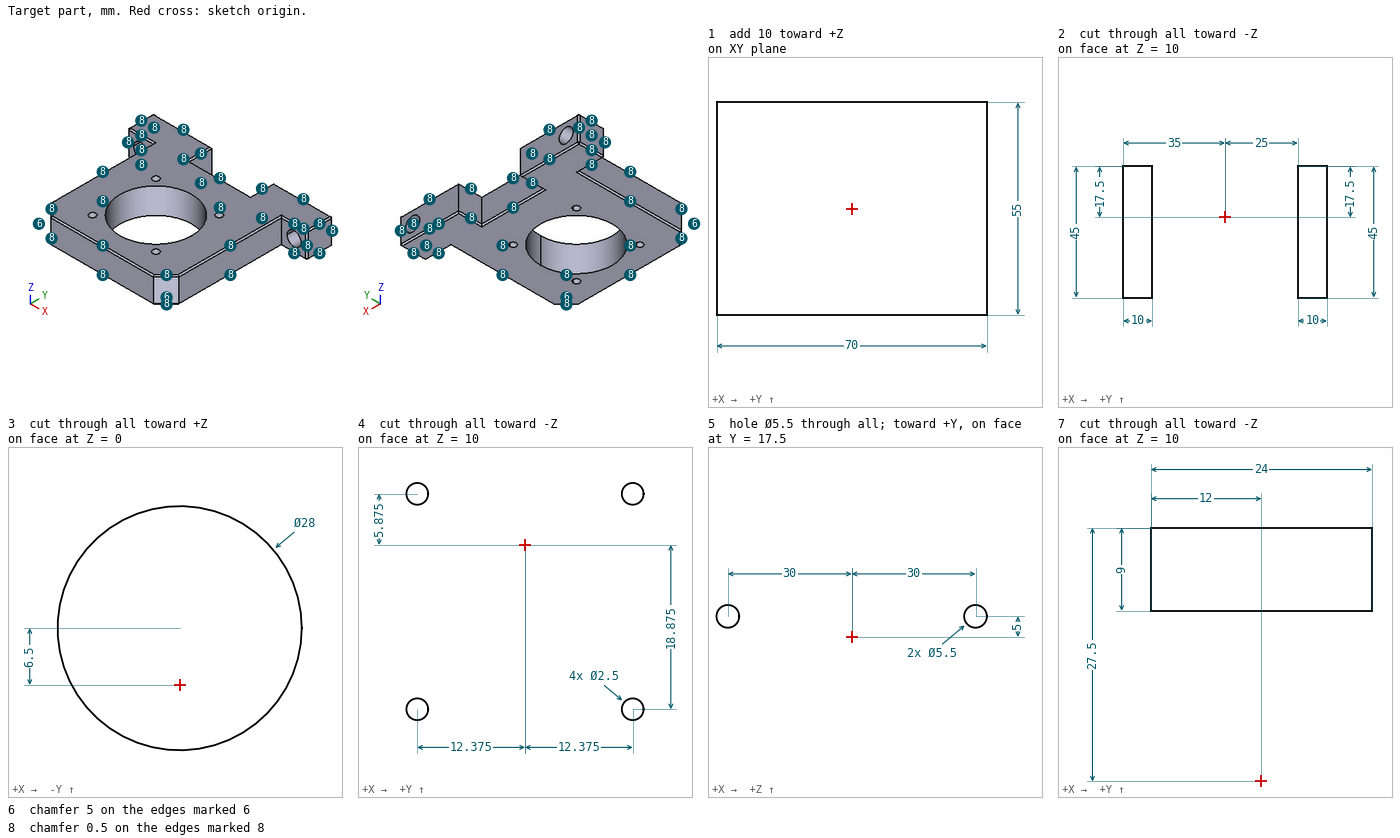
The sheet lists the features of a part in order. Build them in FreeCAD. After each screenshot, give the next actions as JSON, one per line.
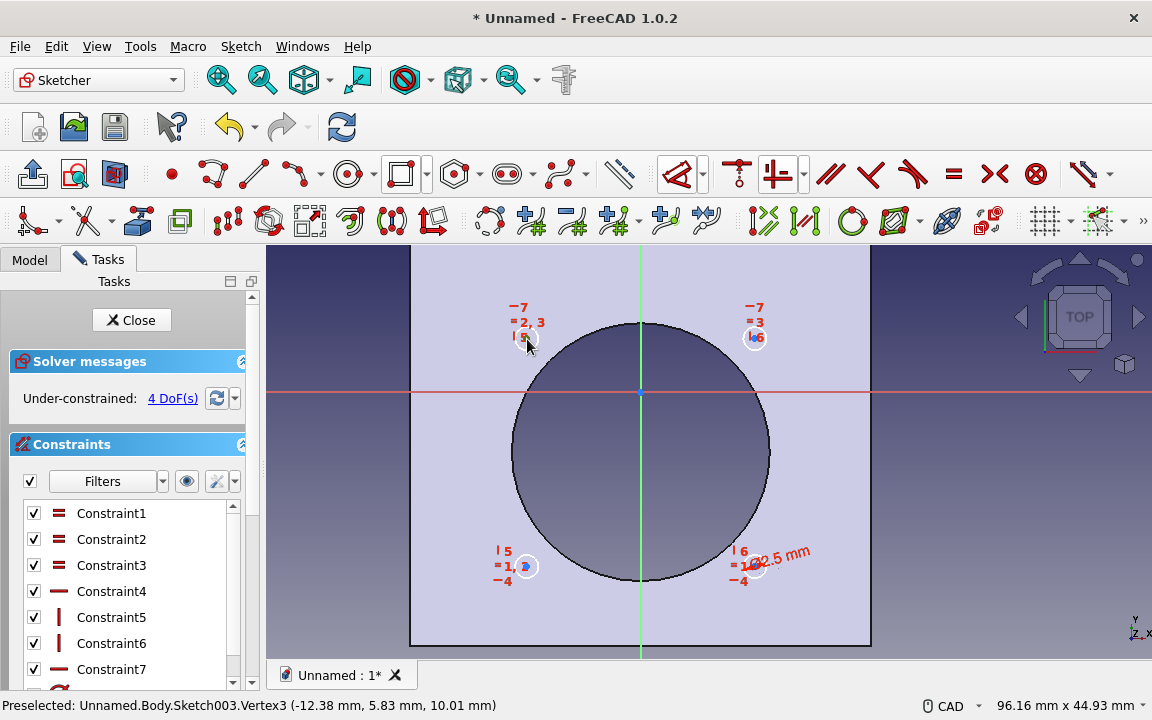
{"action": "key", "text": "i"}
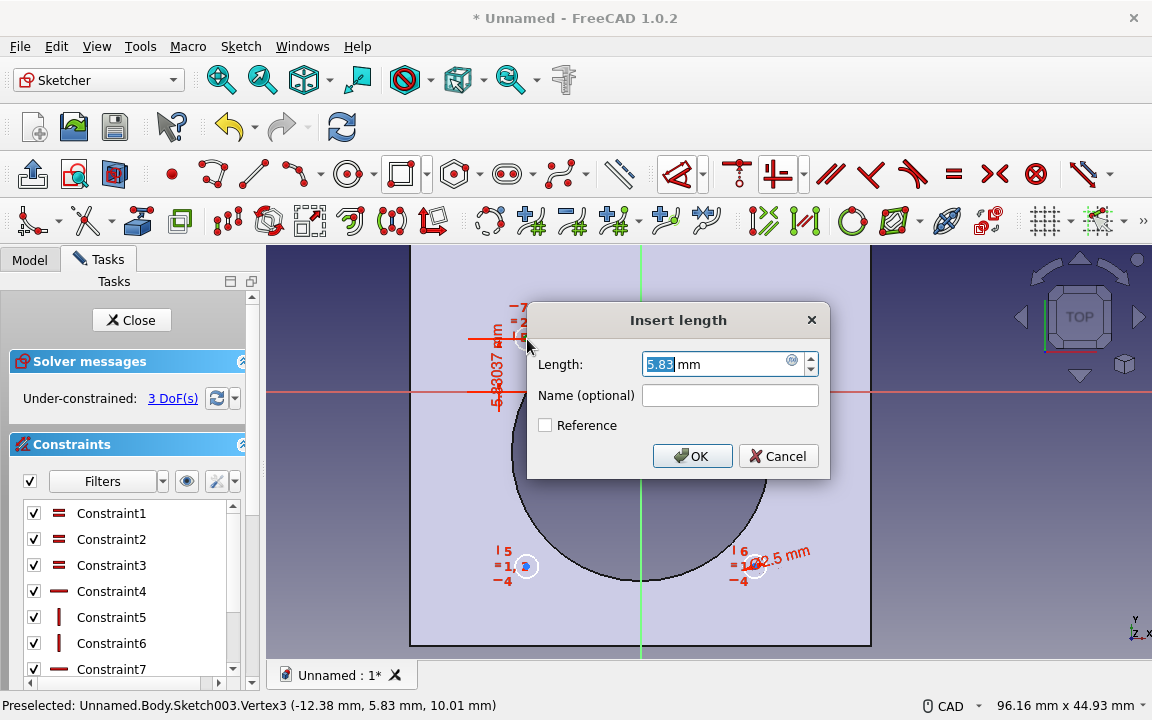
{"action": "type", "text": "5.875"}
{"action": "key", "text": "Return"}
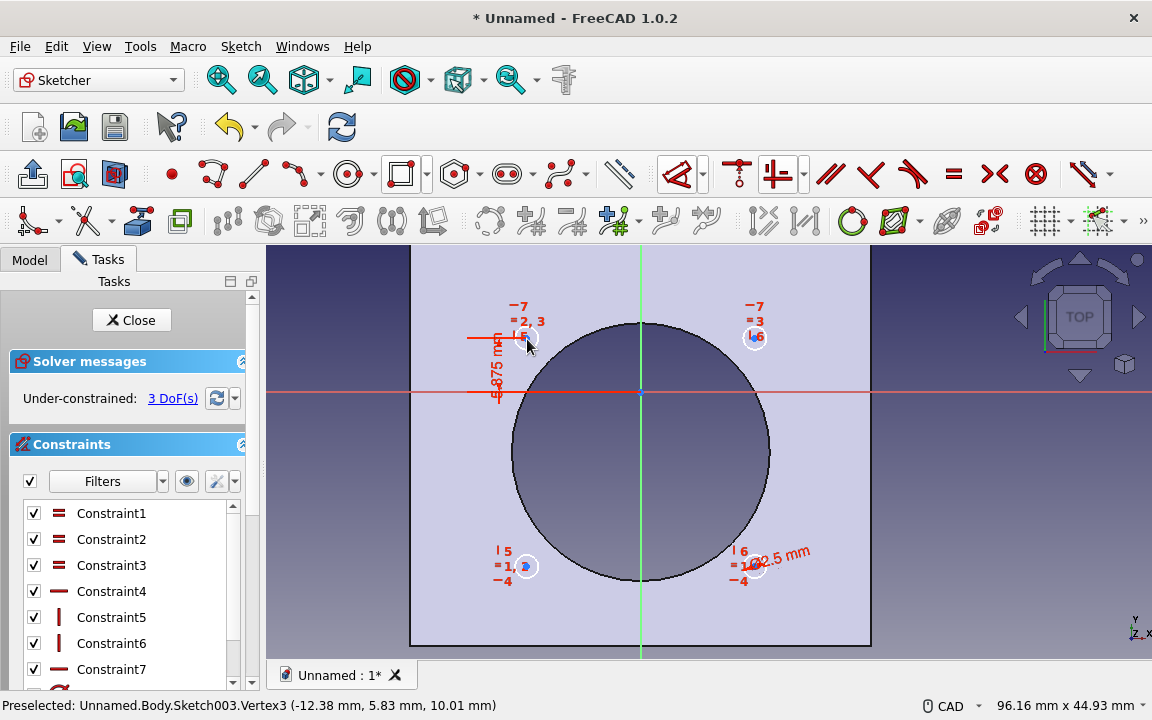
{"action": "left_click", "coordinate": [755, 567]}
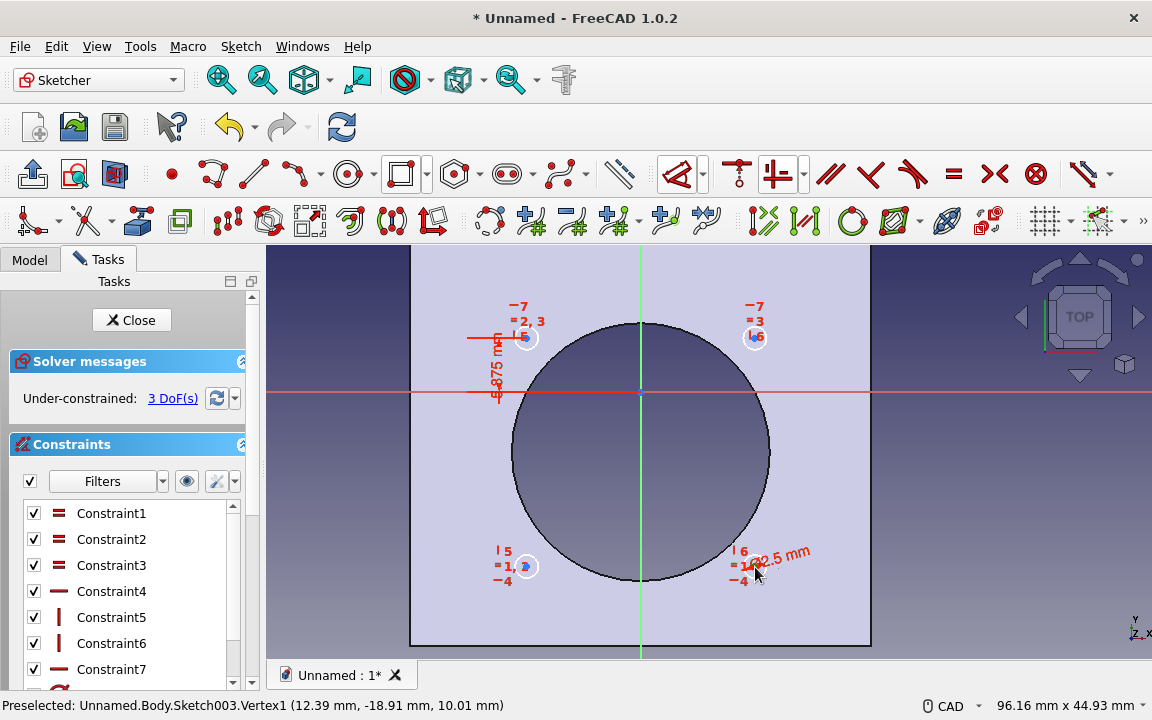
{"action": "left_click", "coordinate": [702, 174]}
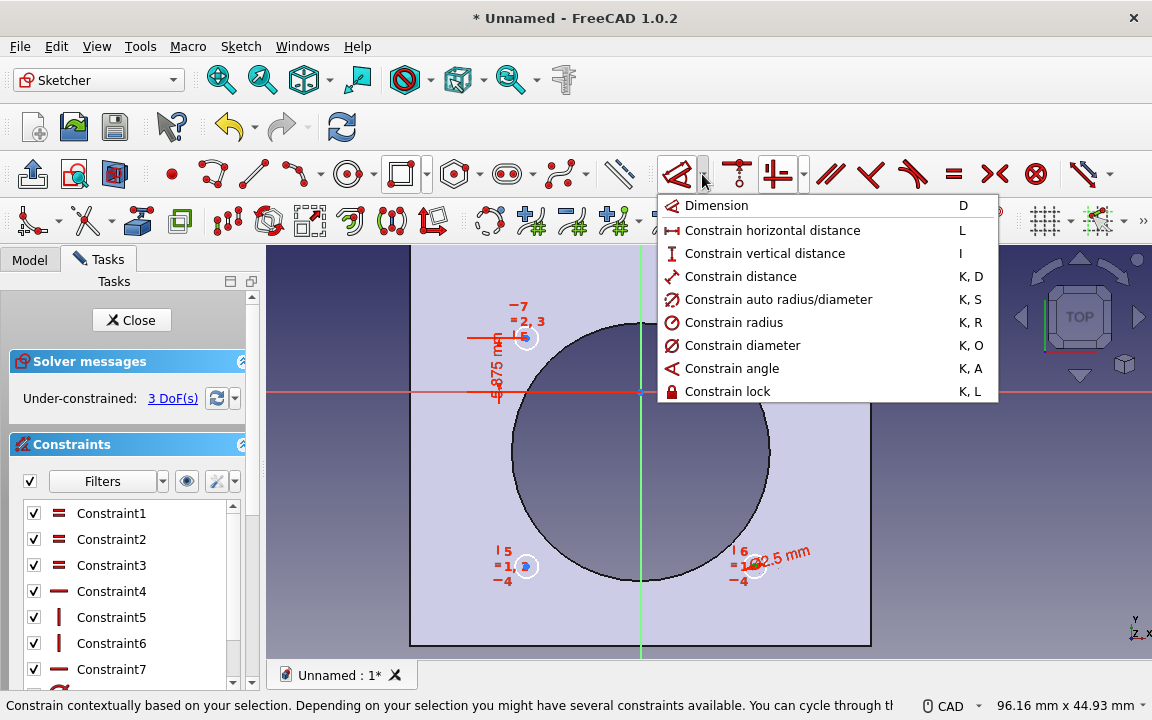
{"action": "left_click", "coordinate": [828, 230]}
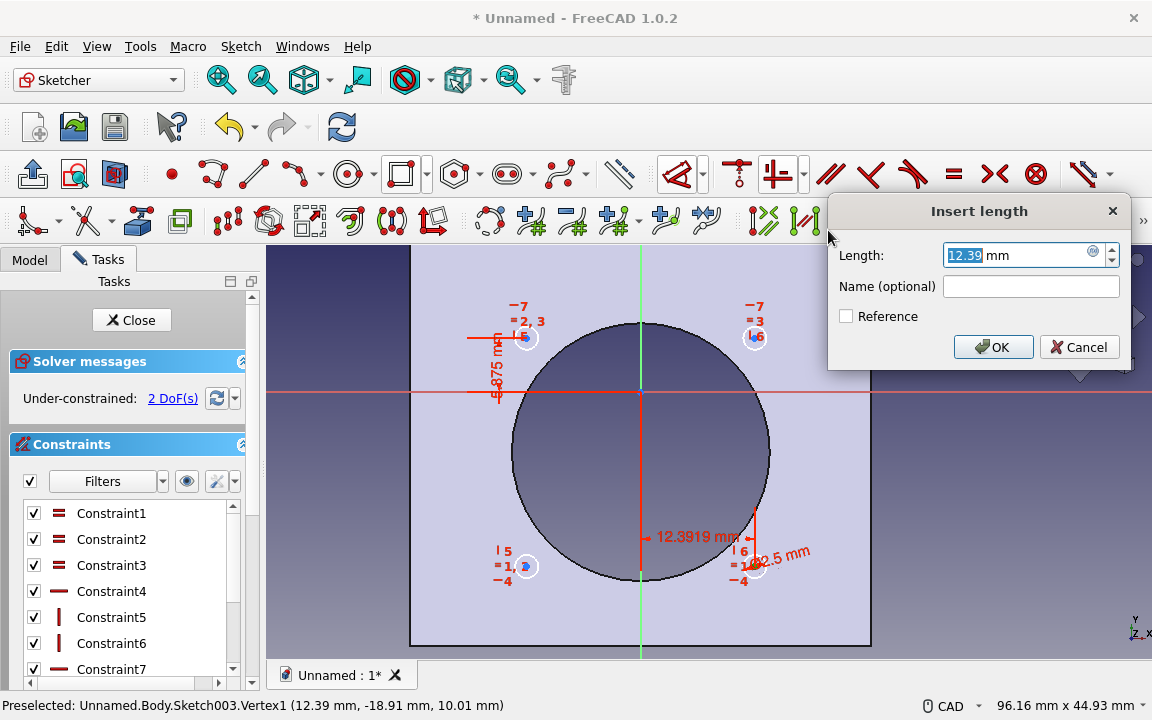
{"action": "type", "text": "12.375"}
{"action": "key", "text": "Return"}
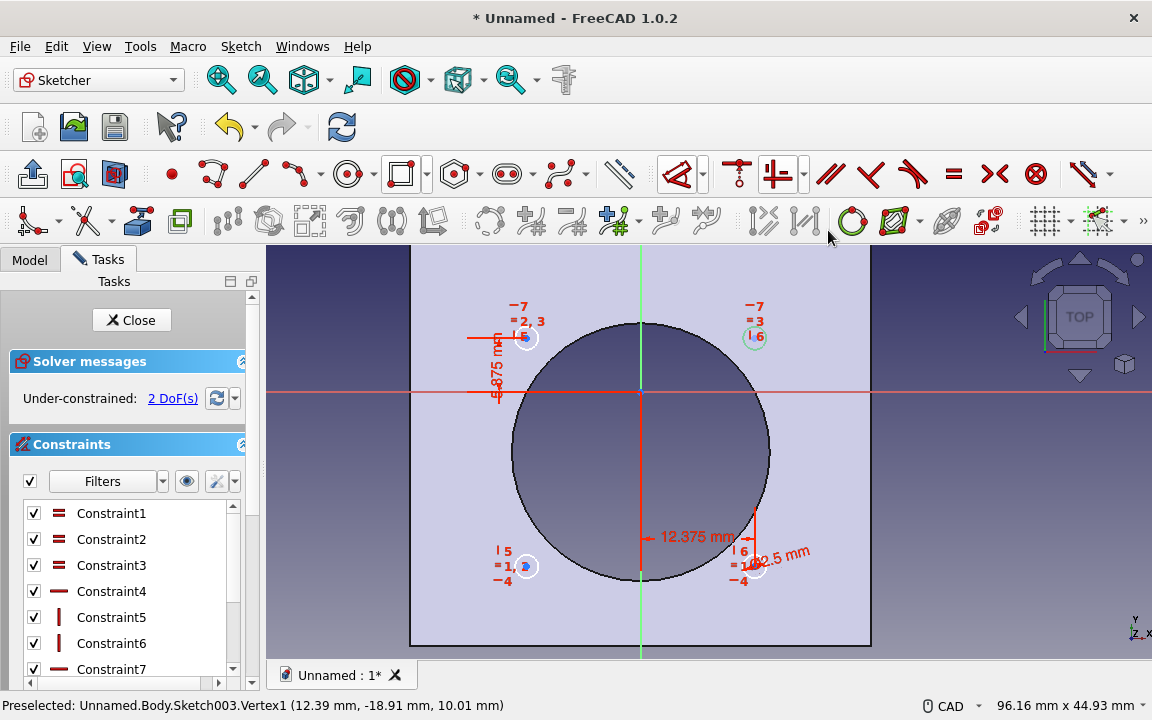
{"action": "left_click", "coordinate": [755, 567]}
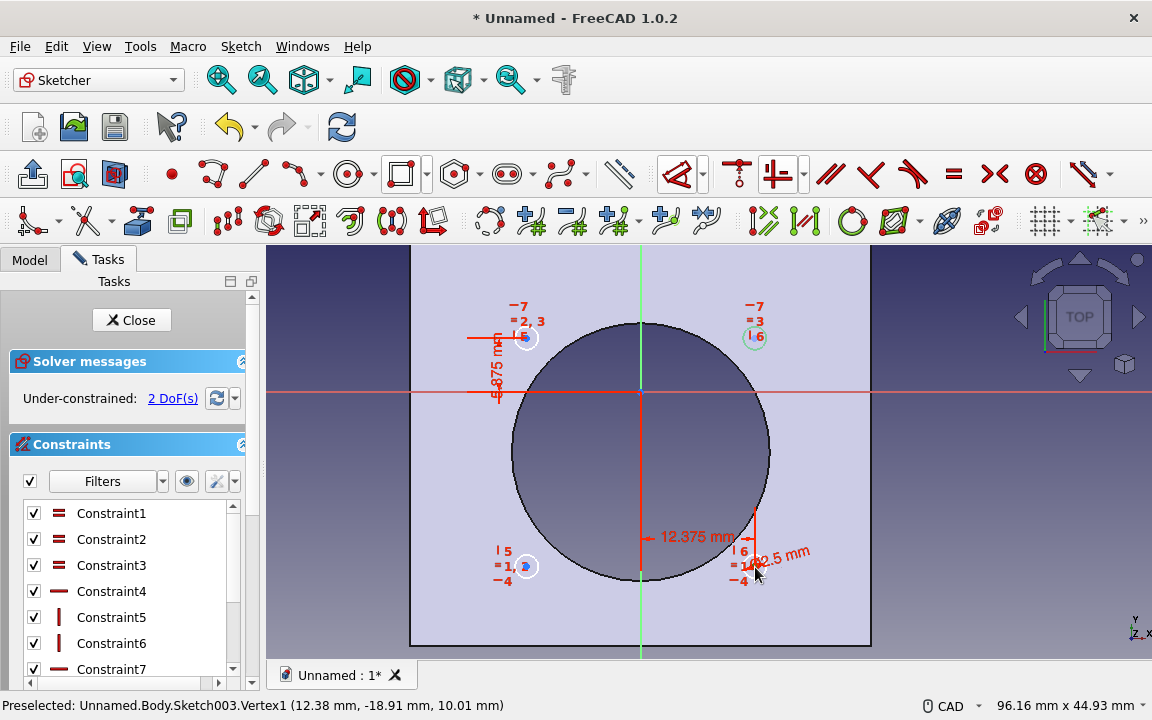
{"action": "left_click", "coordinate": [702, 174]}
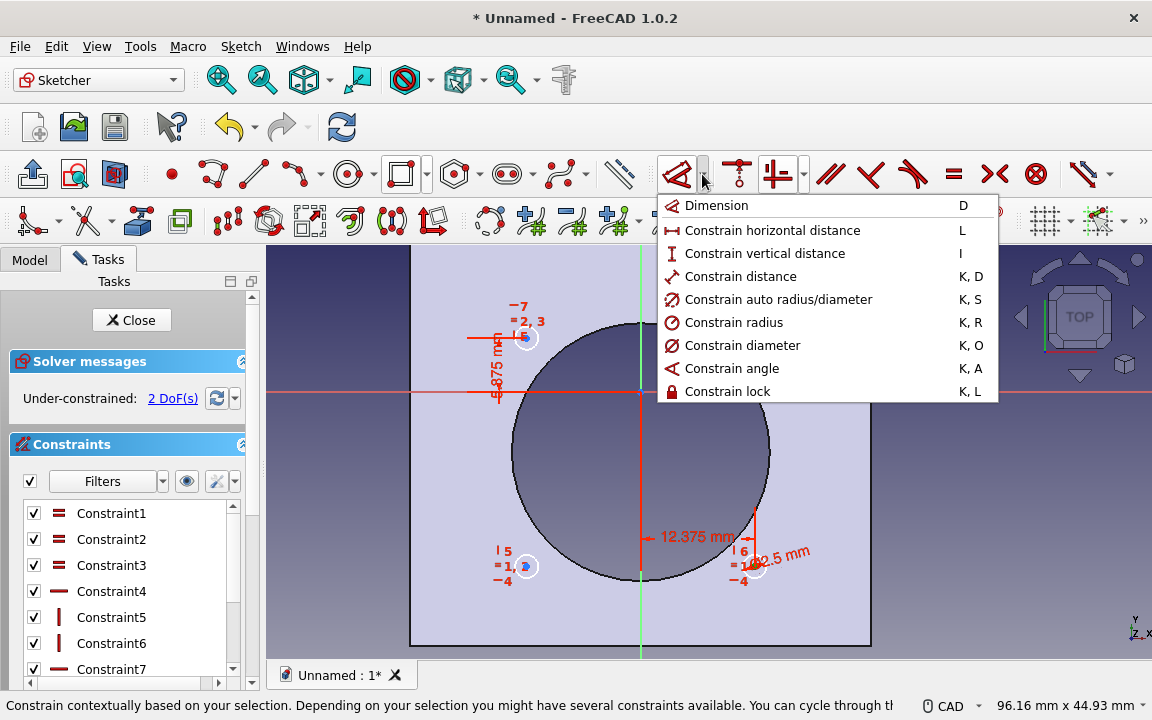
{"action": "left_click", "coordinate": [828, 254]}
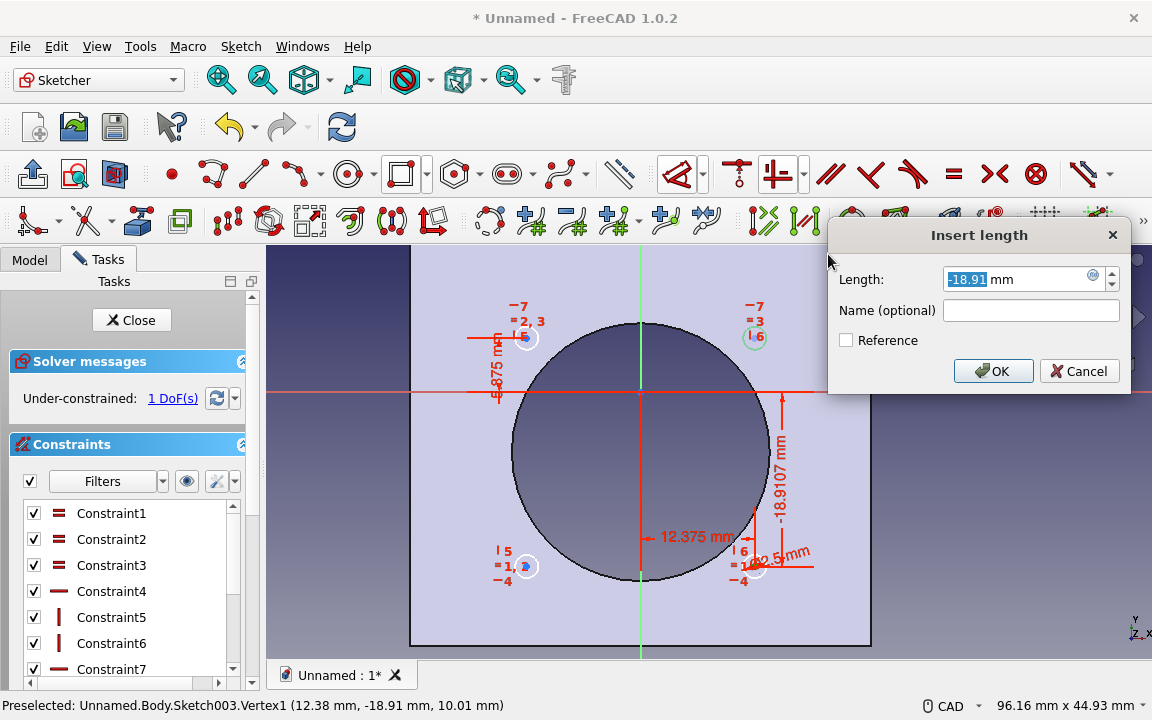
{"action": "type", "text": "-18.875"}
{"action": "key", "text": "Return"}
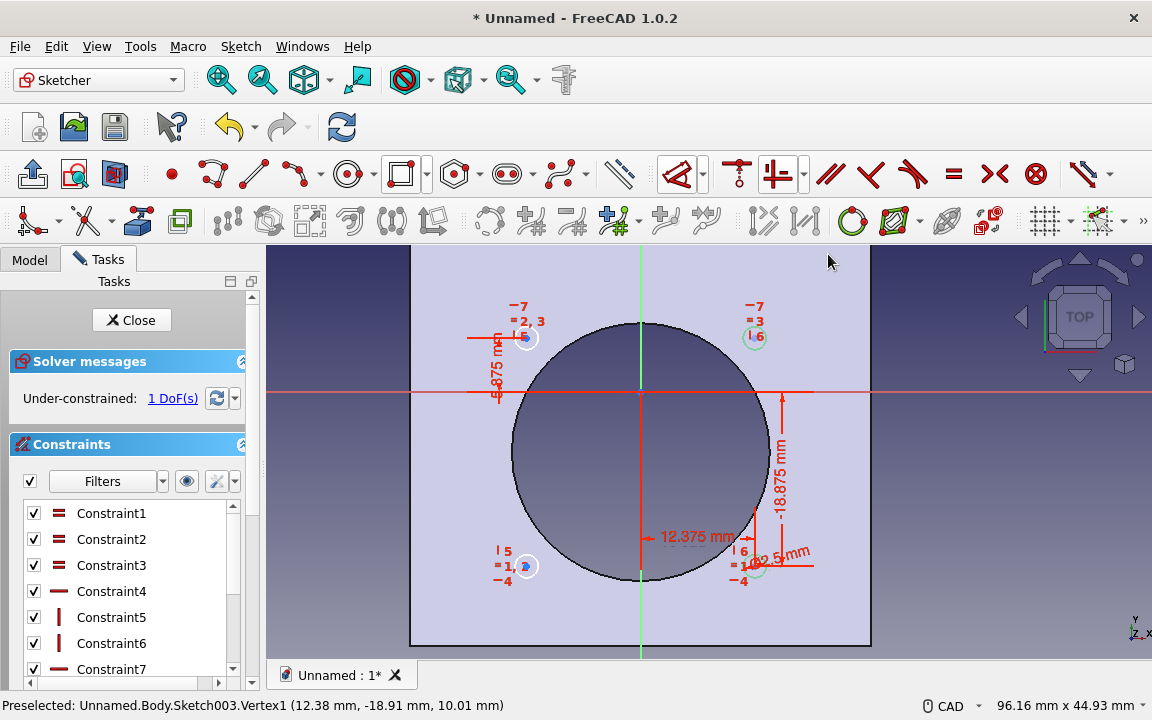
{"action": "left_click", "coordinate": [527, 566]}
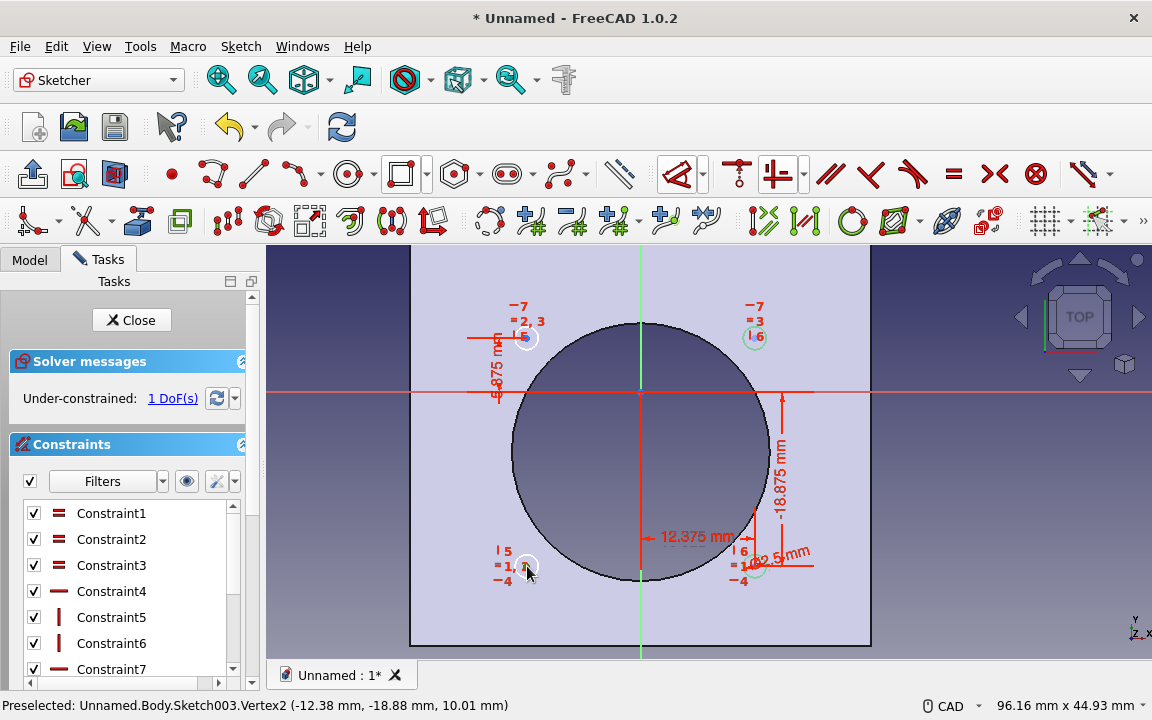
{"action": "left_click", "coordinate": [702, 174]}